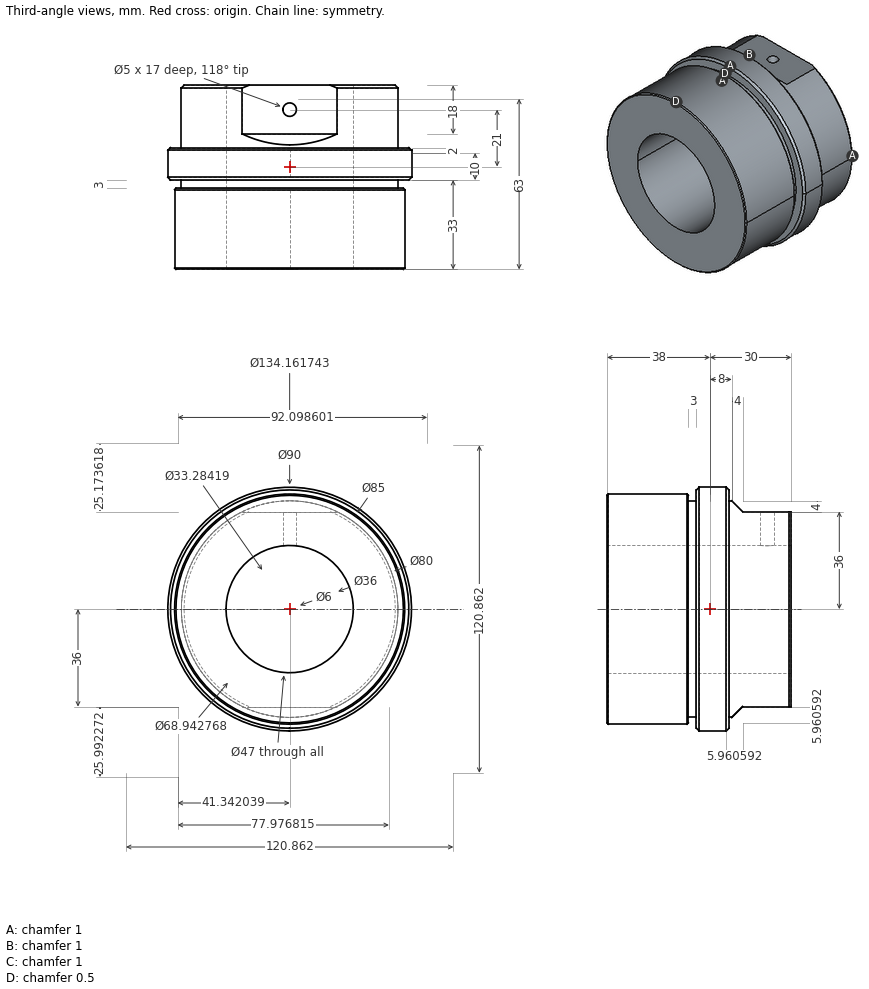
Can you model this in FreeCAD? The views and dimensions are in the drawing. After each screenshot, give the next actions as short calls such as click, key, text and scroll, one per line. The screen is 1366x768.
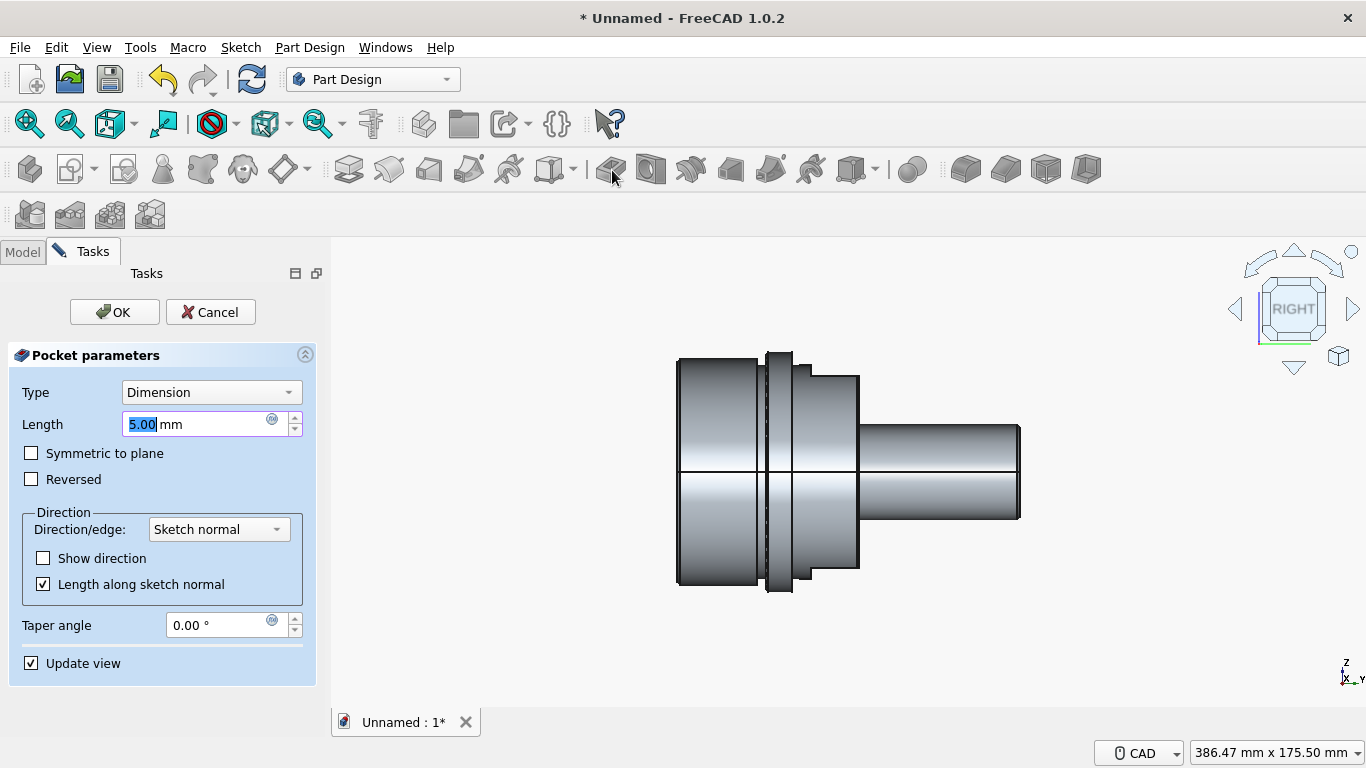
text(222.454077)
key(Tab)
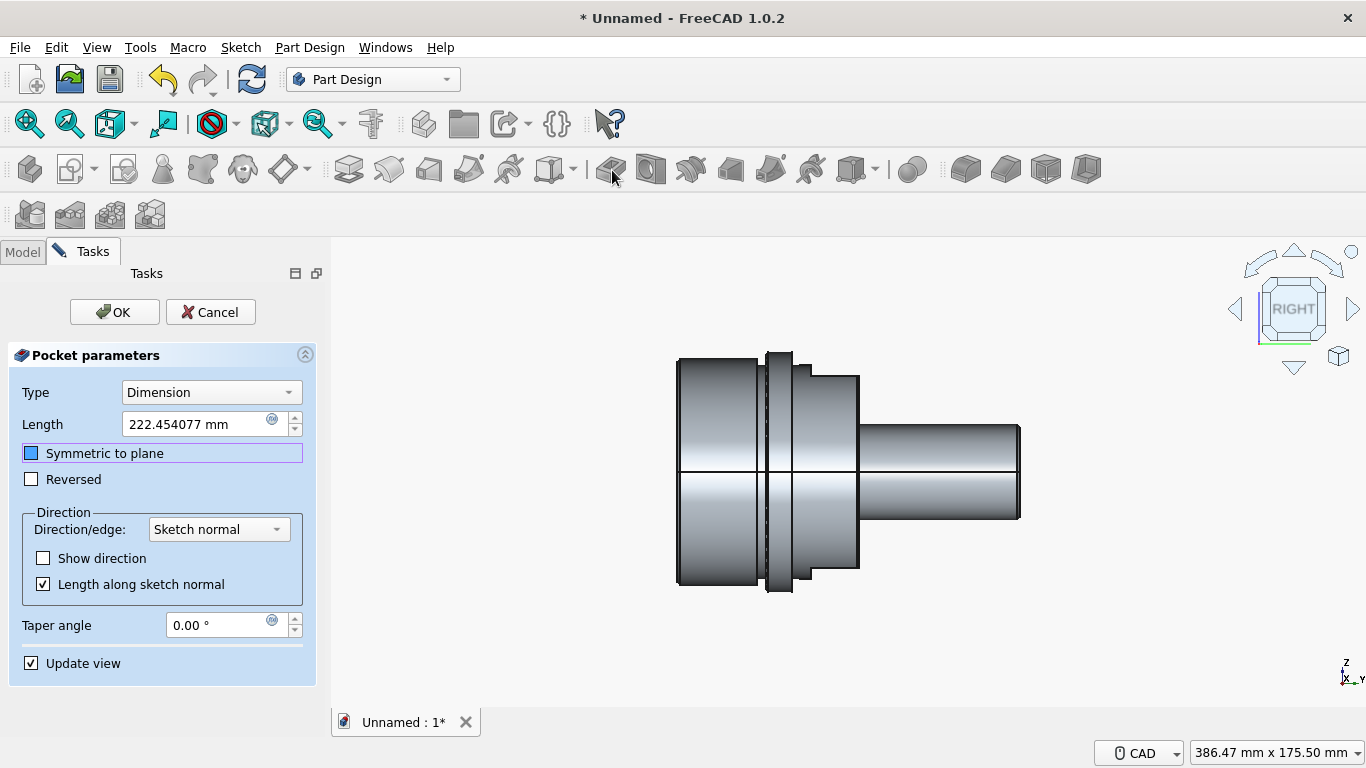
click(30, 453)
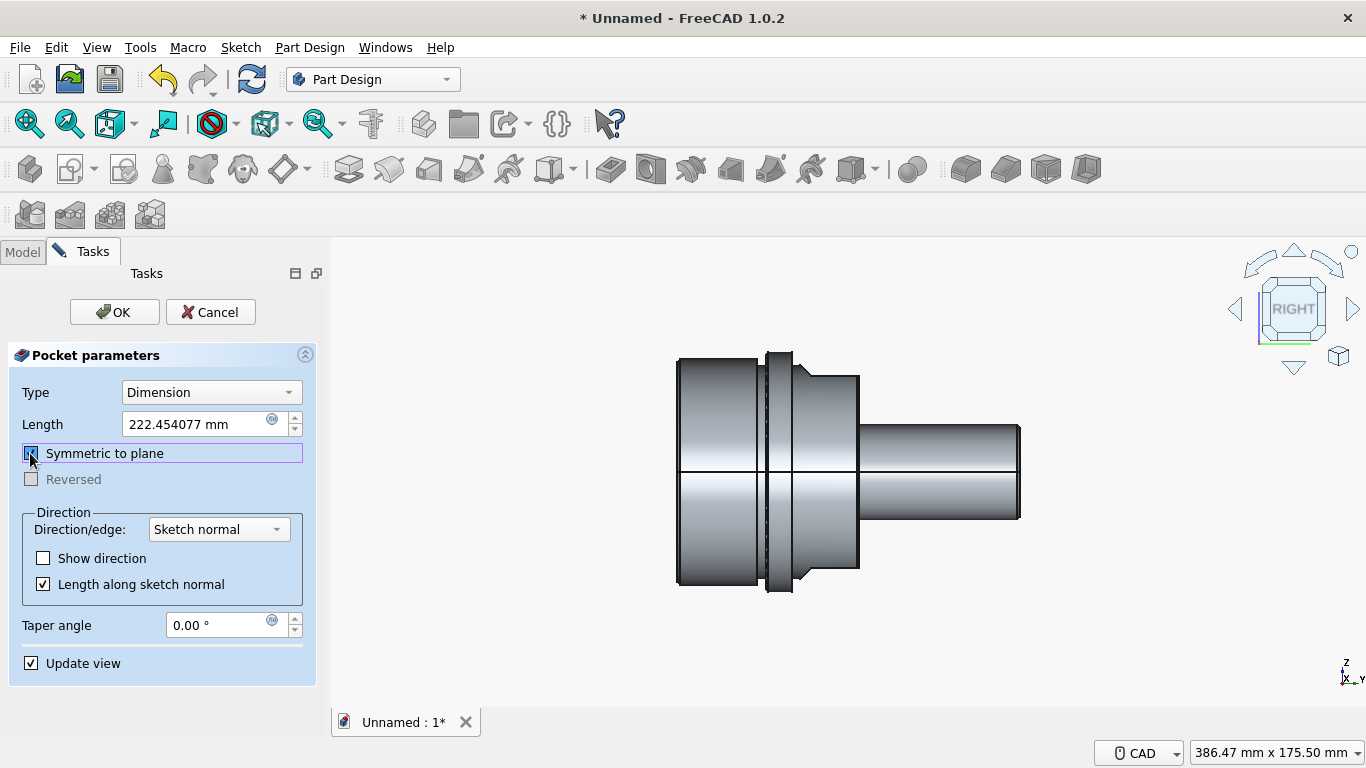
click(115, 312)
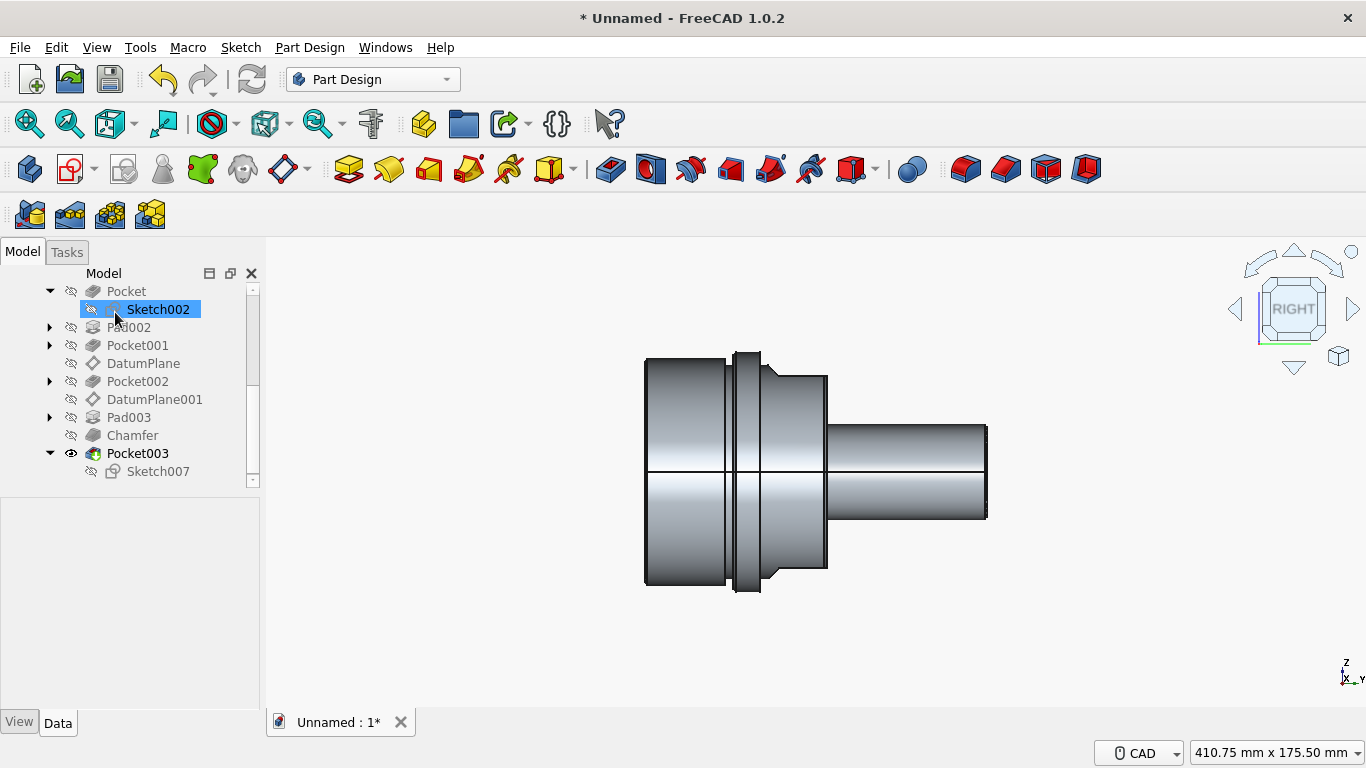
key(4)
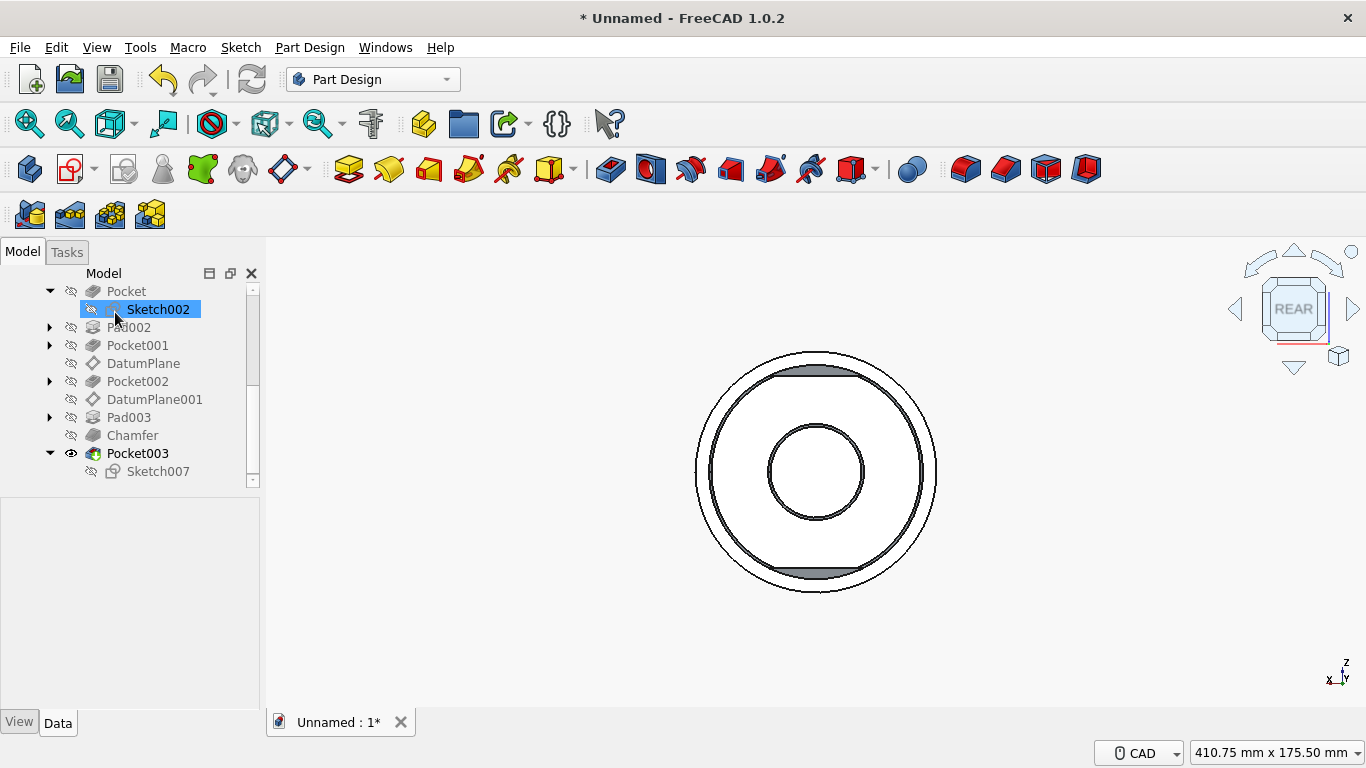
scroll(713, 437, up, 10)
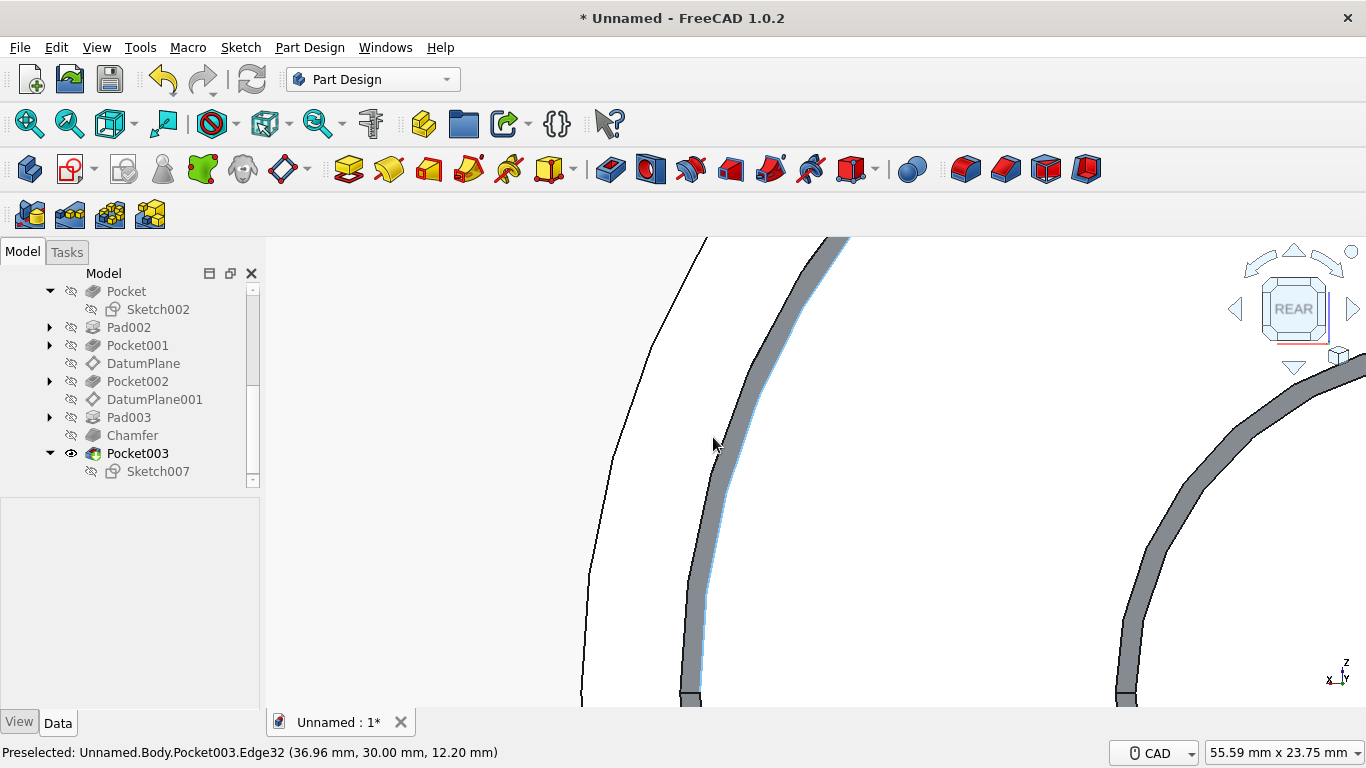
click(709, 438)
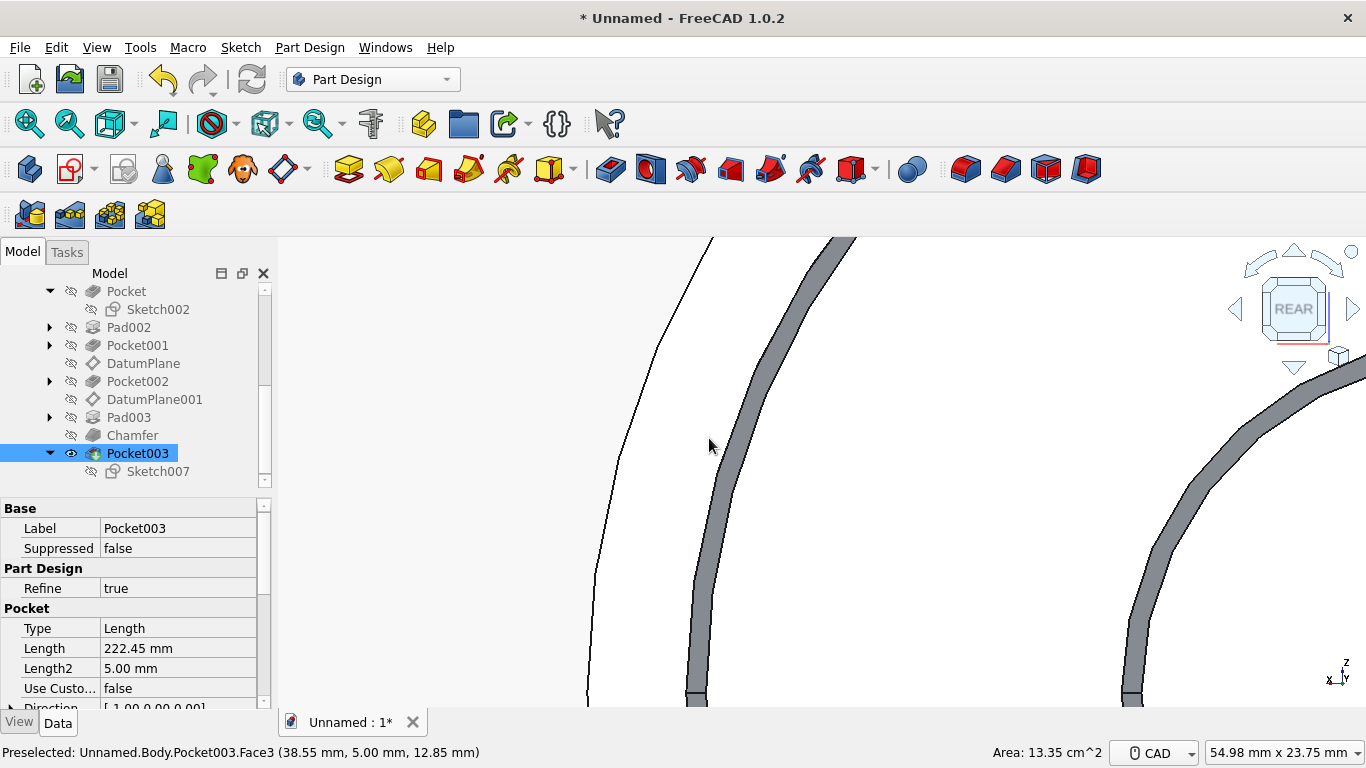
click(70, 170)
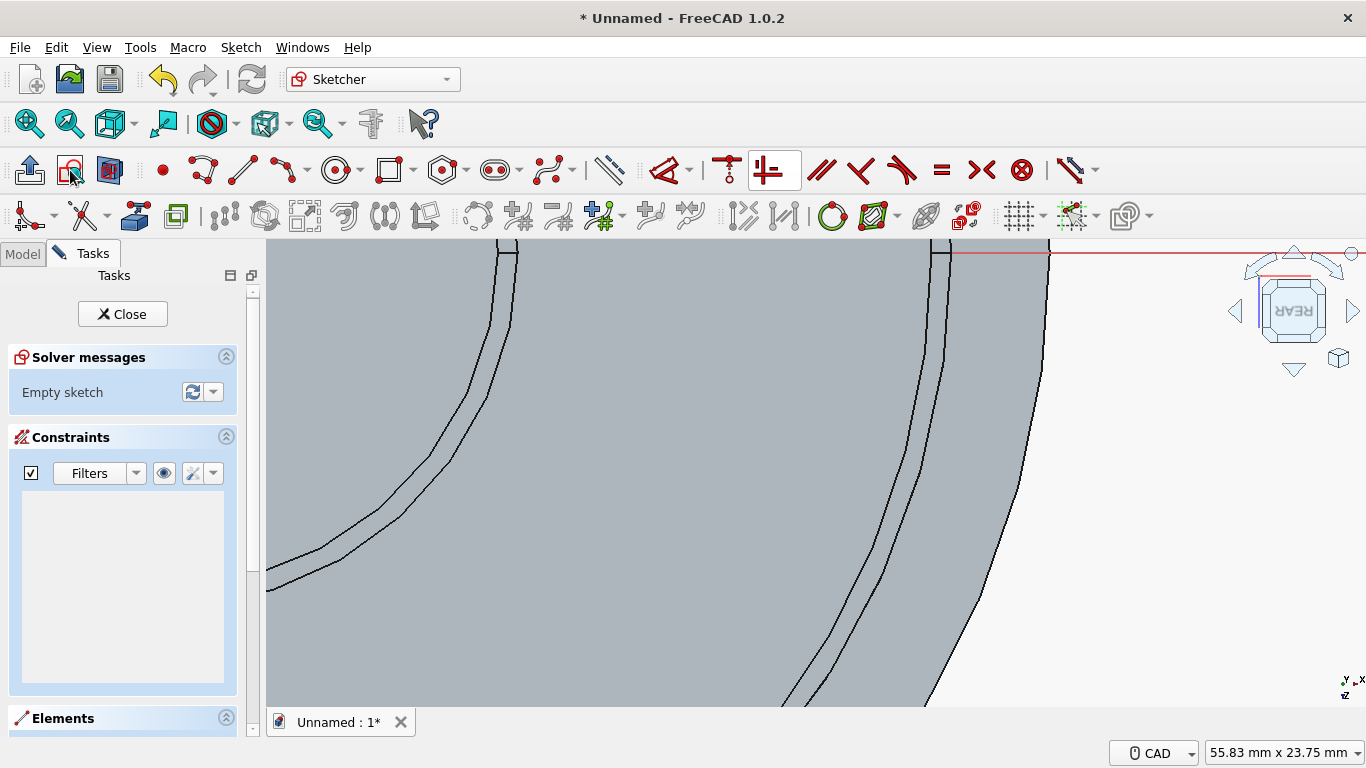
click(110, 170)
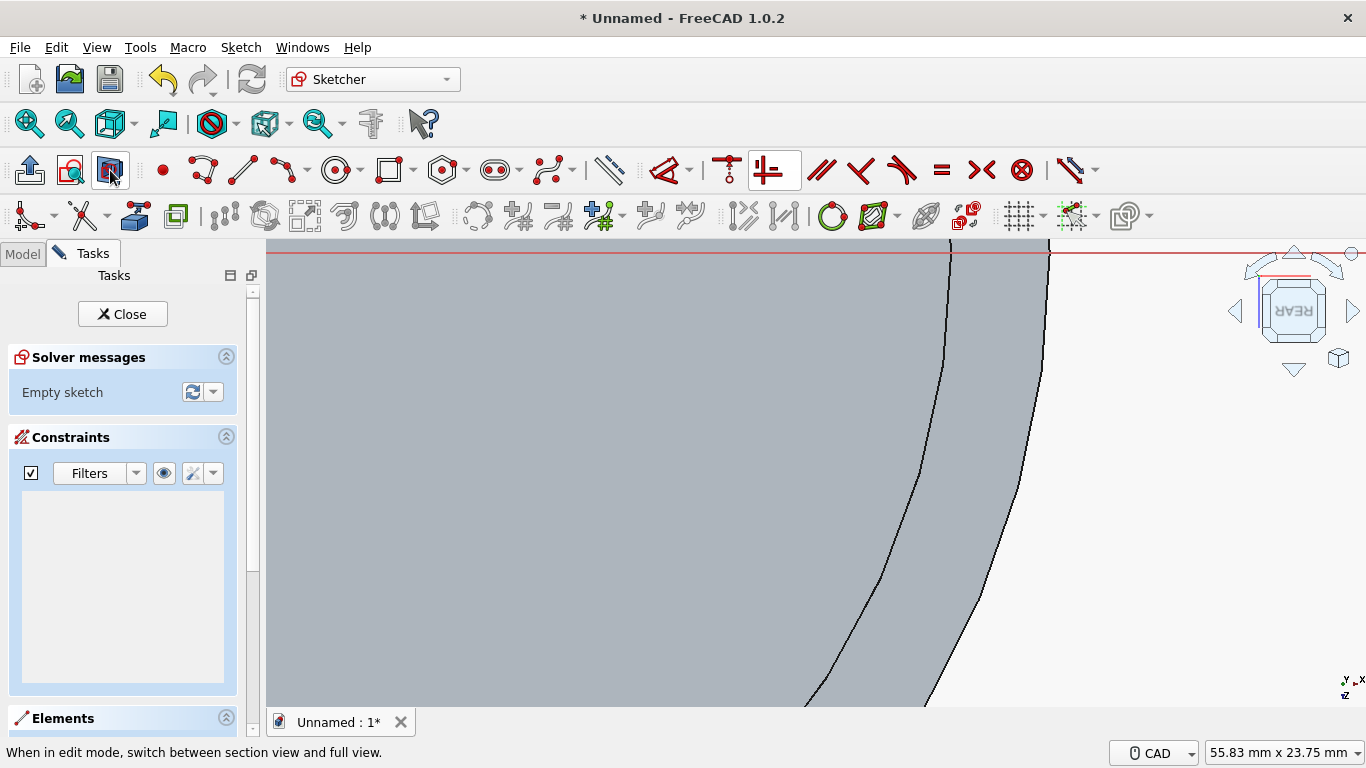
scroll(863, 517, down, 9)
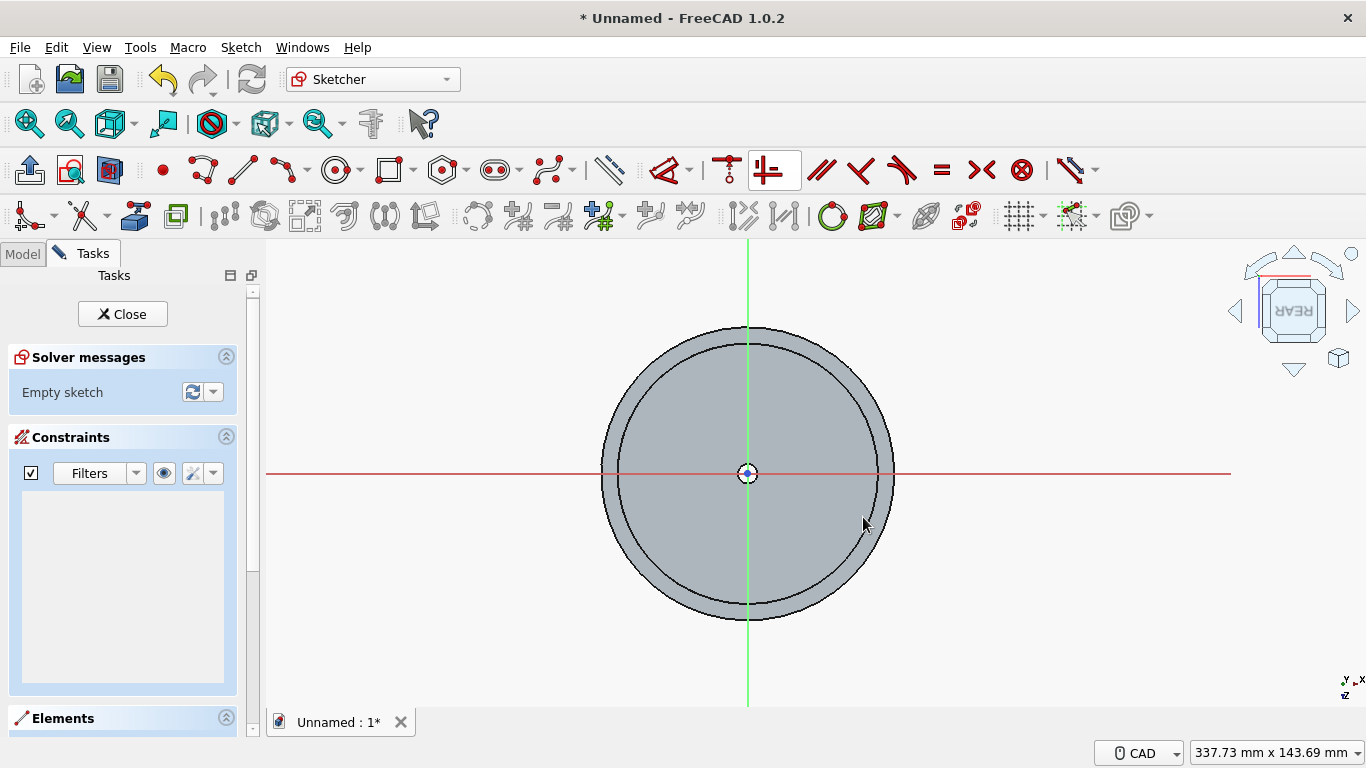
click(336, 170)